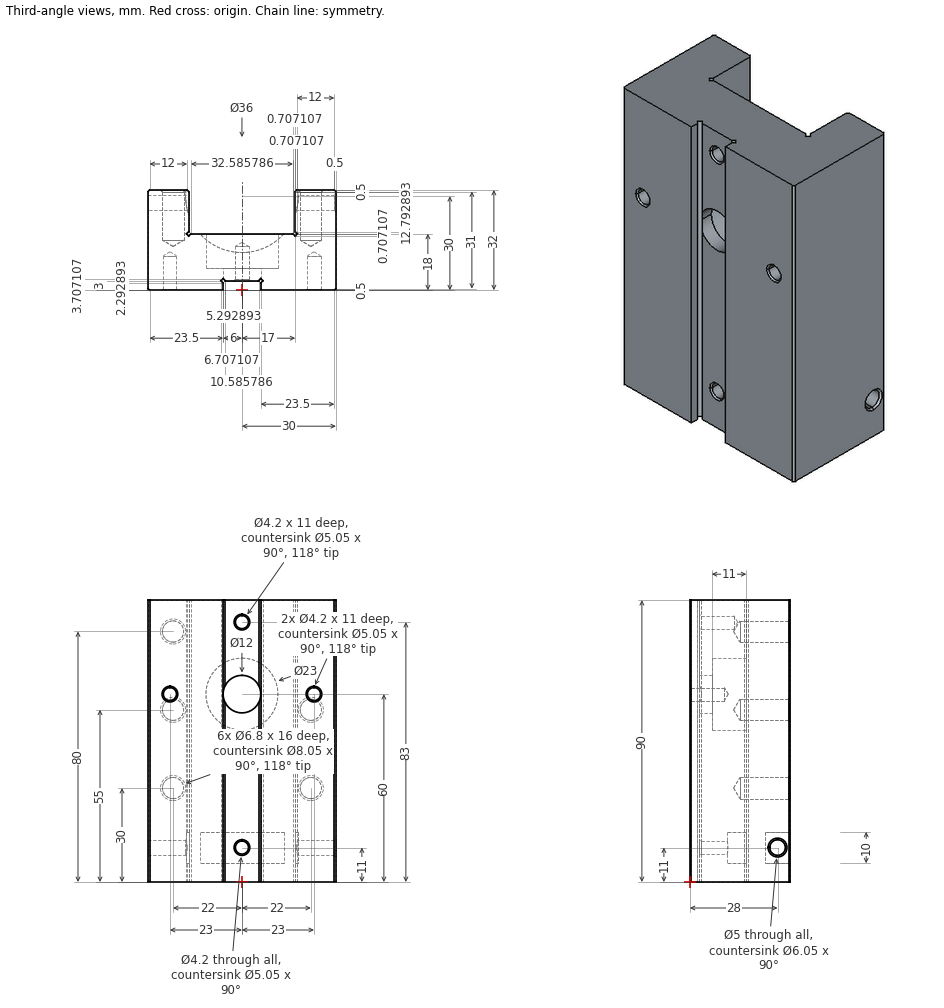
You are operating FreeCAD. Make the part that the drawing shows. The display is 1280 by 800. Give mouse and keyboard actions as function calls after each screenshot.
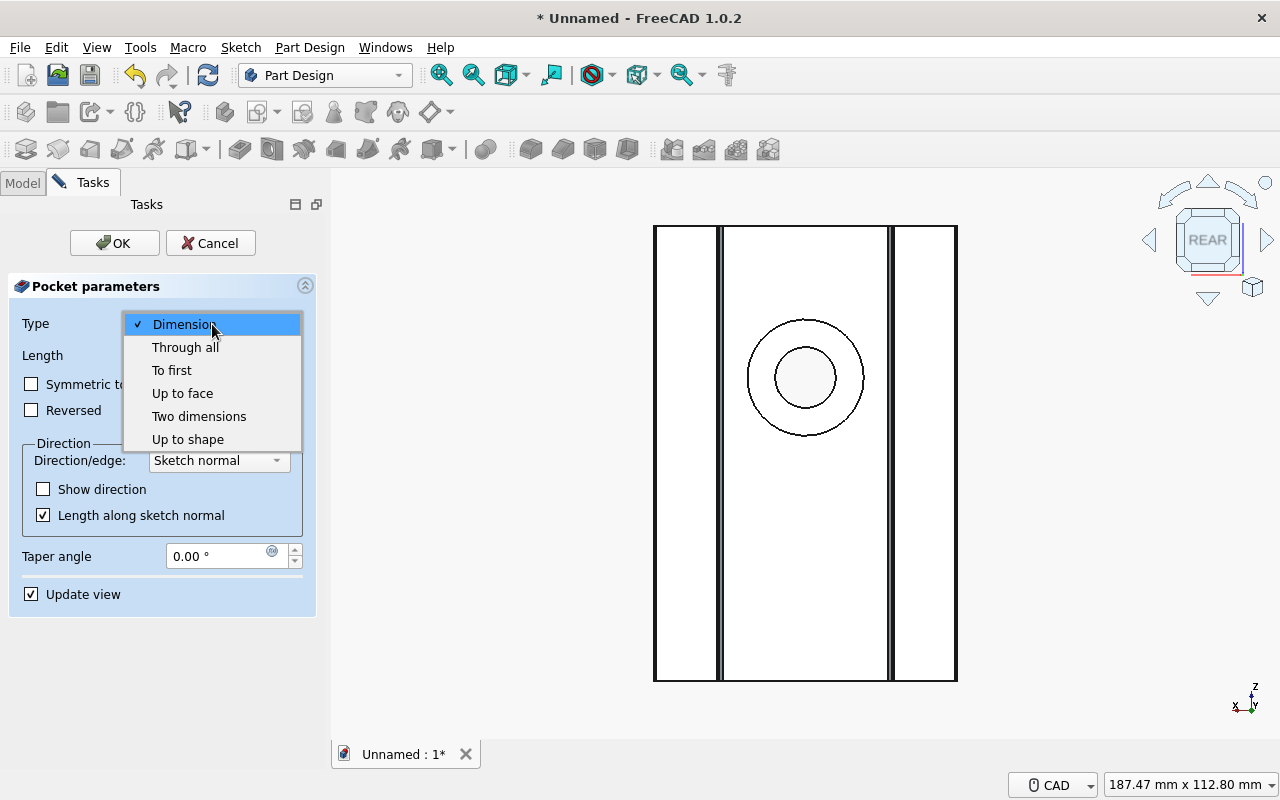
click(212, 348)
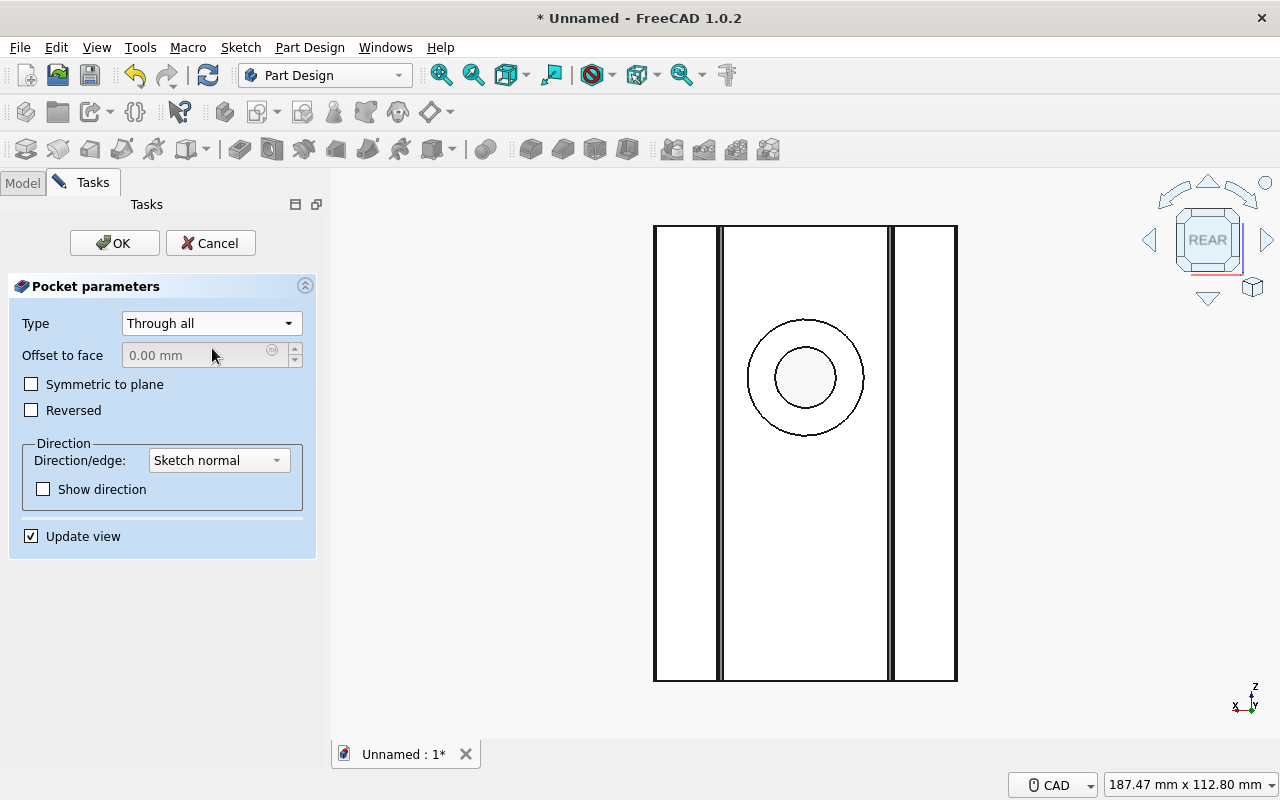
click(115, 243)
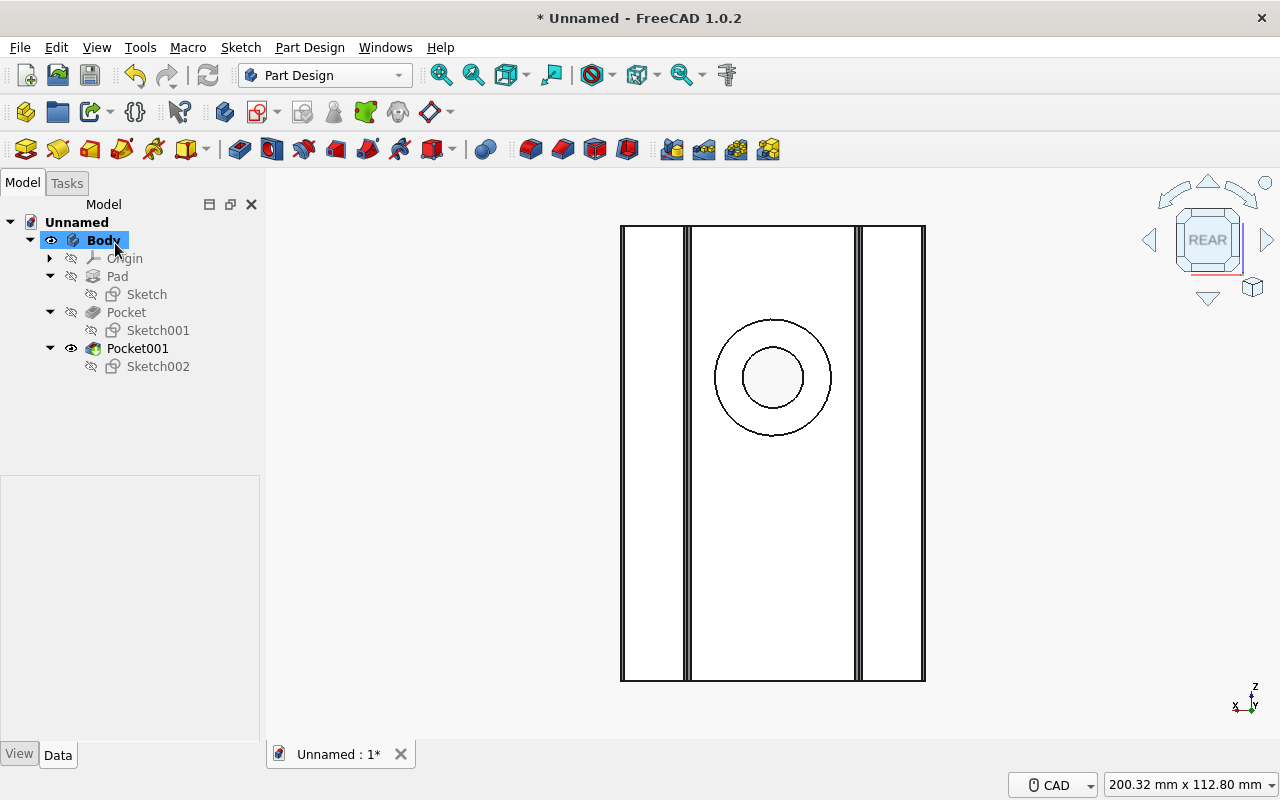
click(50, 258)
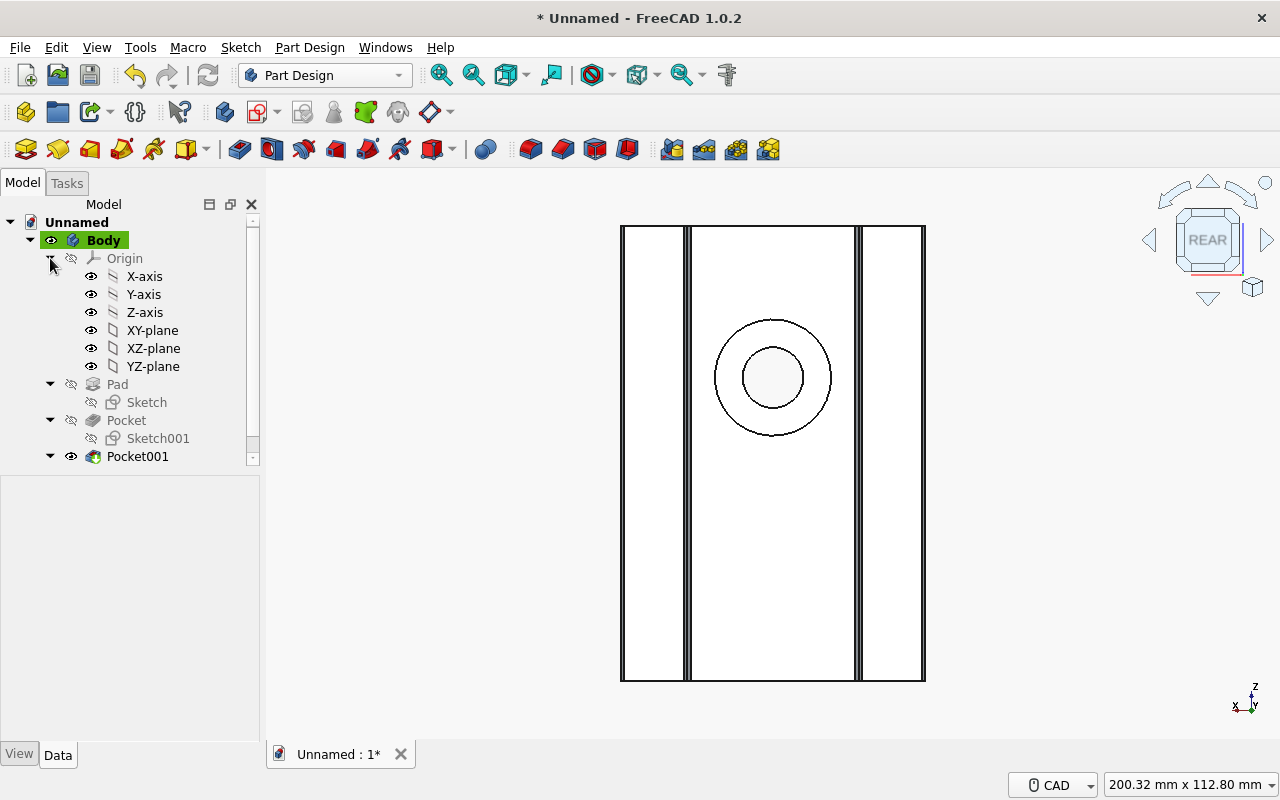
click(136, 330)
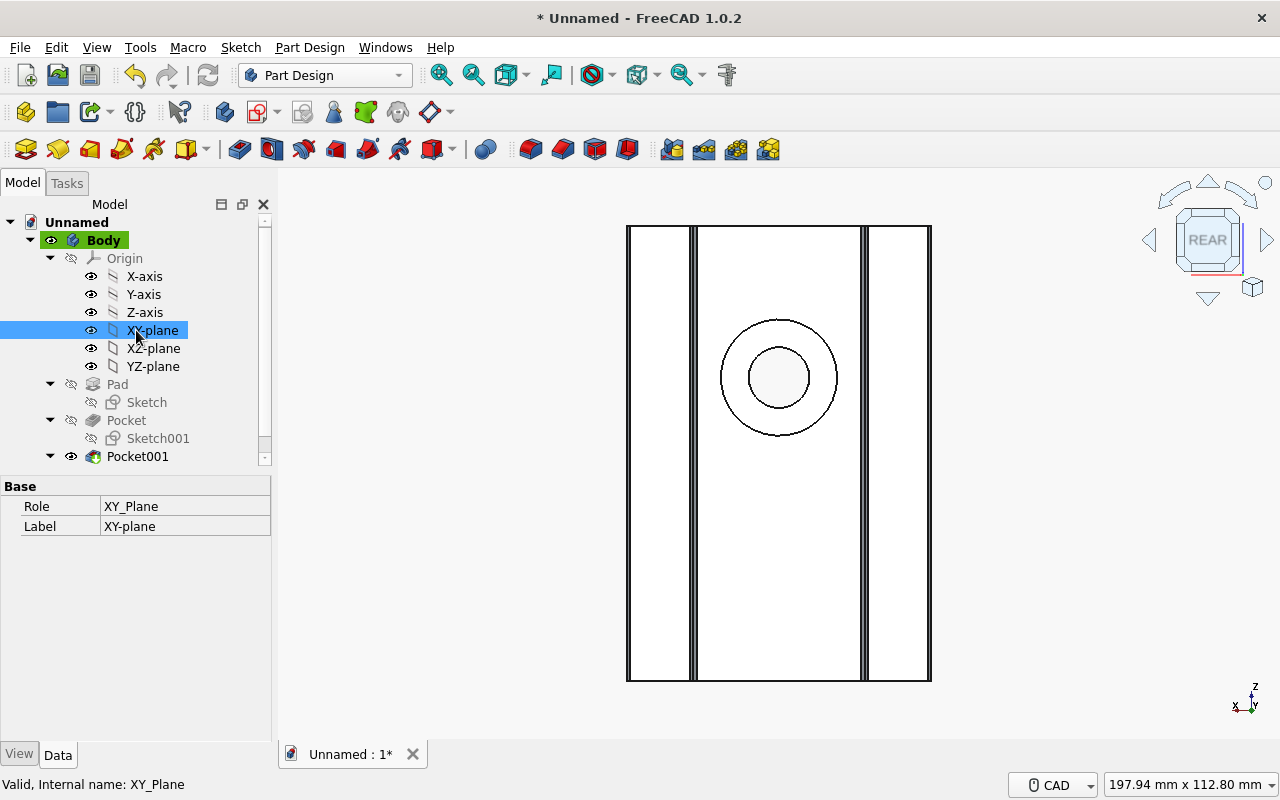
click(430, 112)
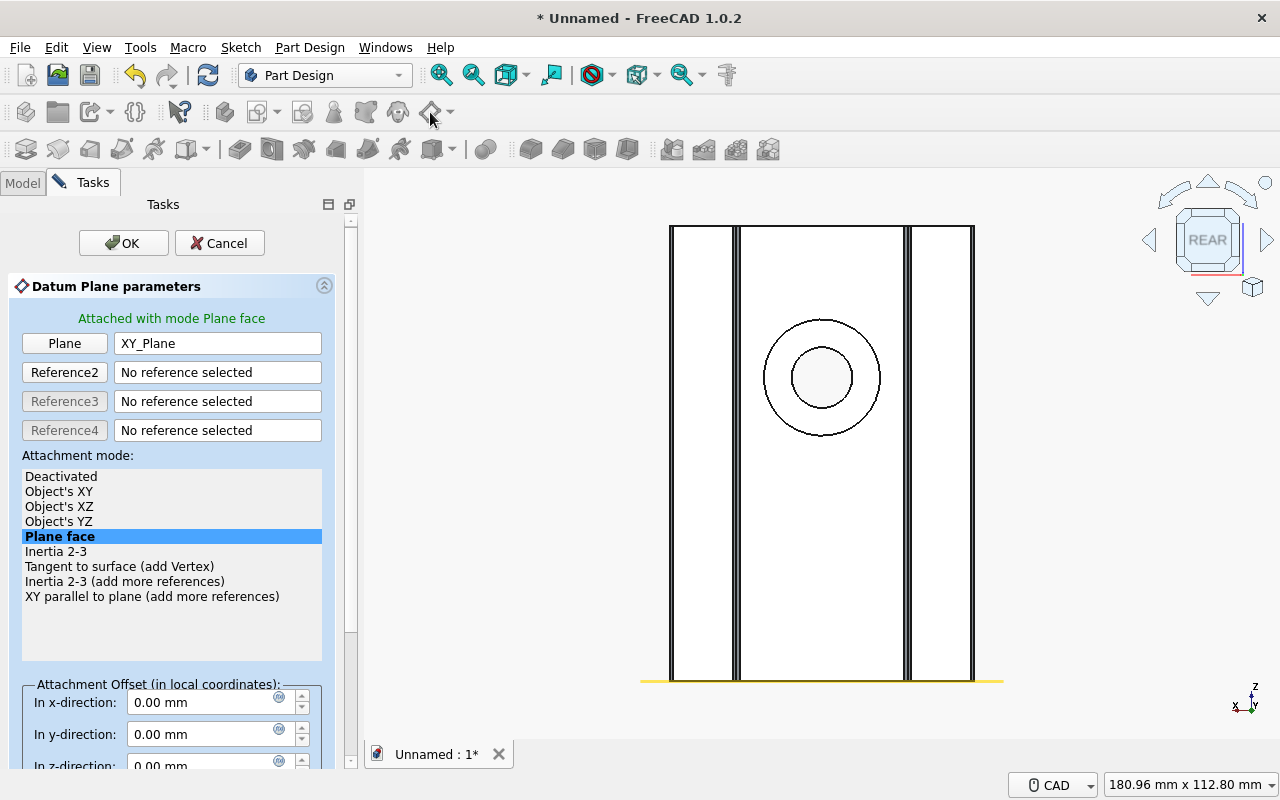
scroll(351, 491, down, 2)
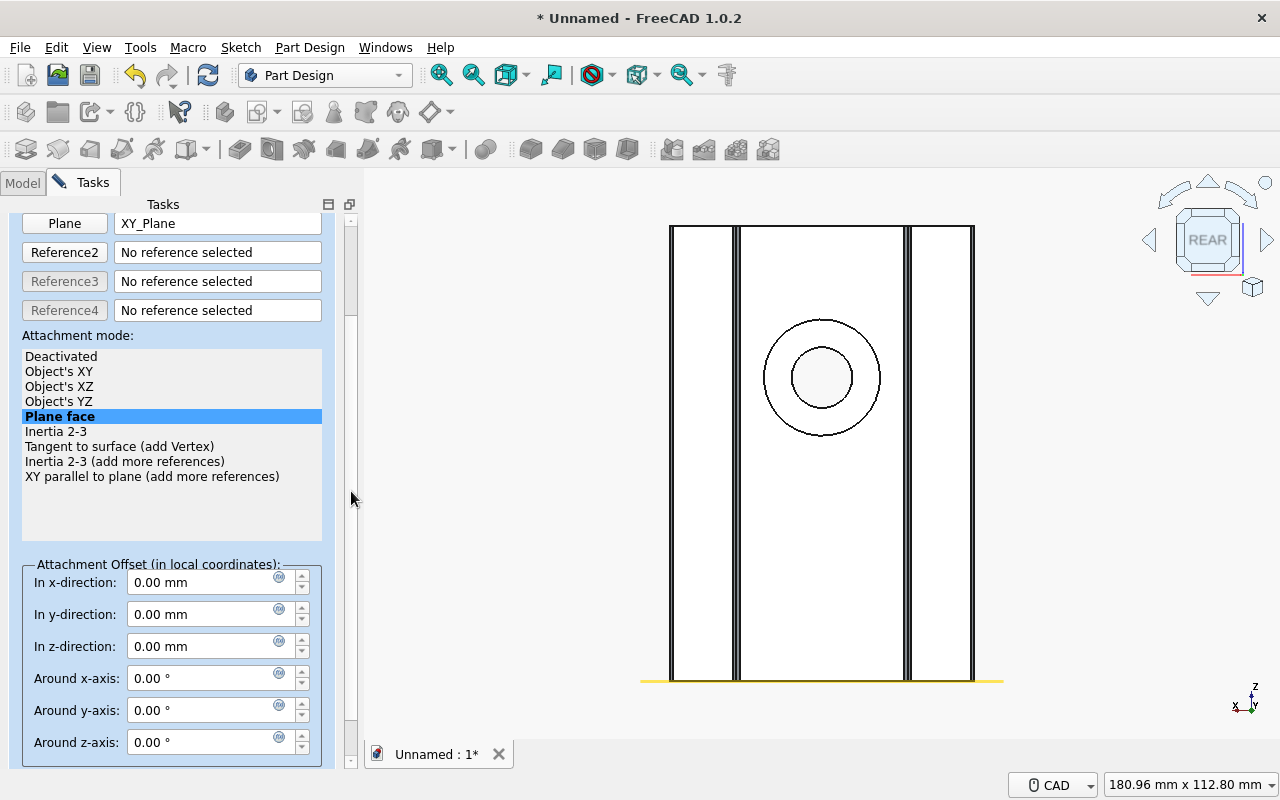
triple_click(210, 646)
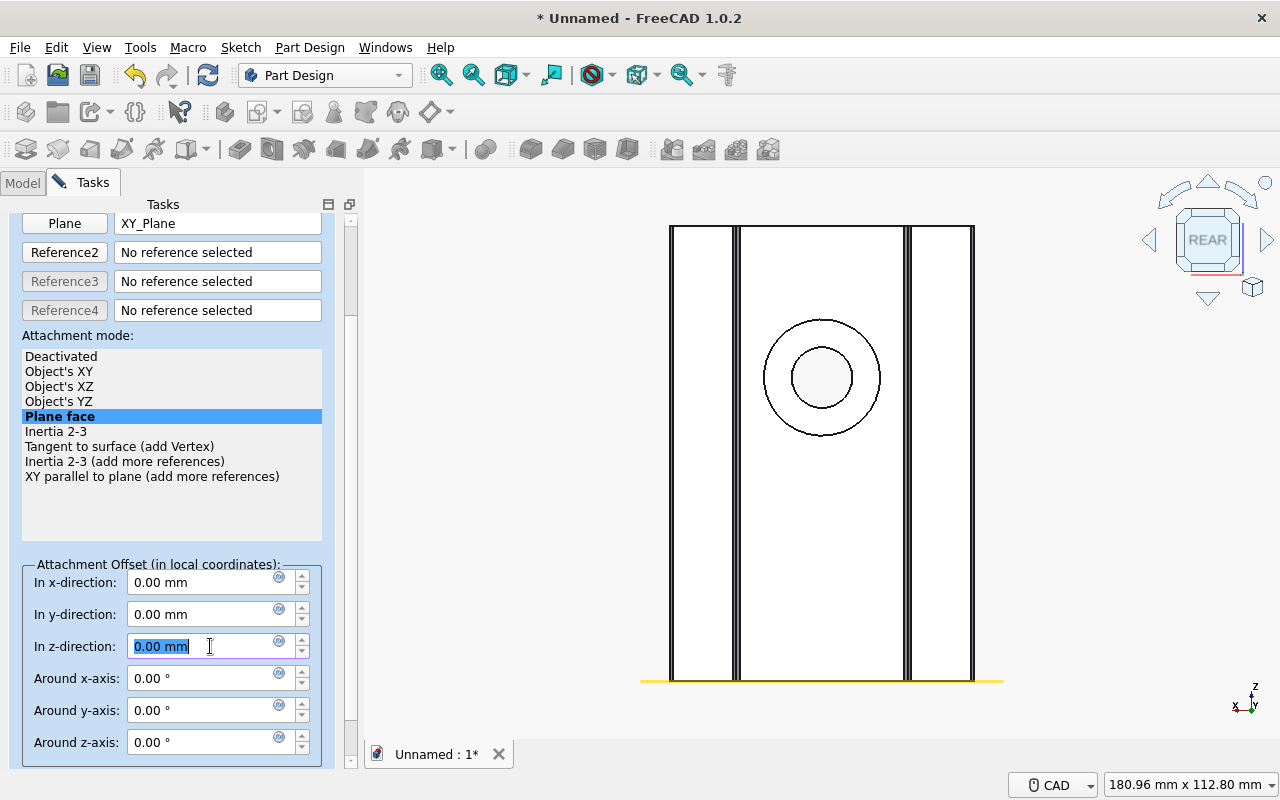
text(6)
key(Tab)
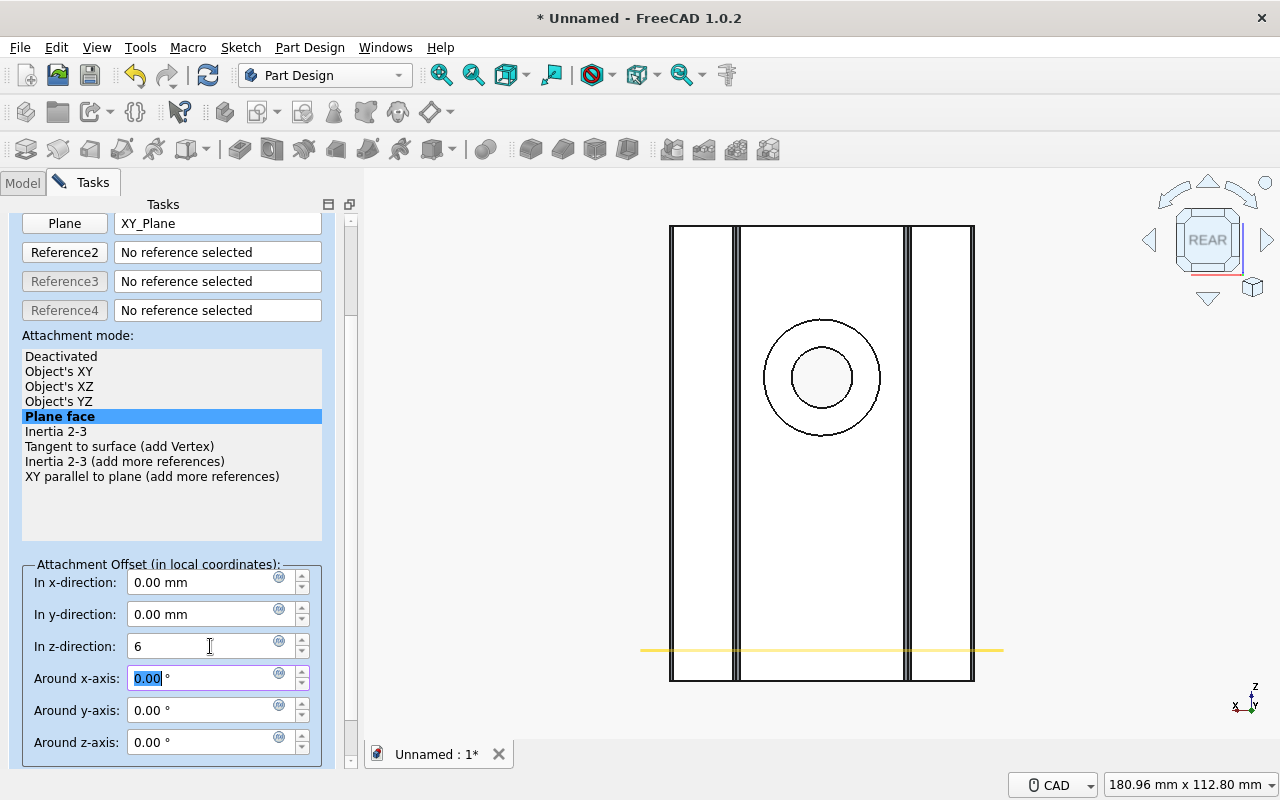
scroll(351, 491, up, 3)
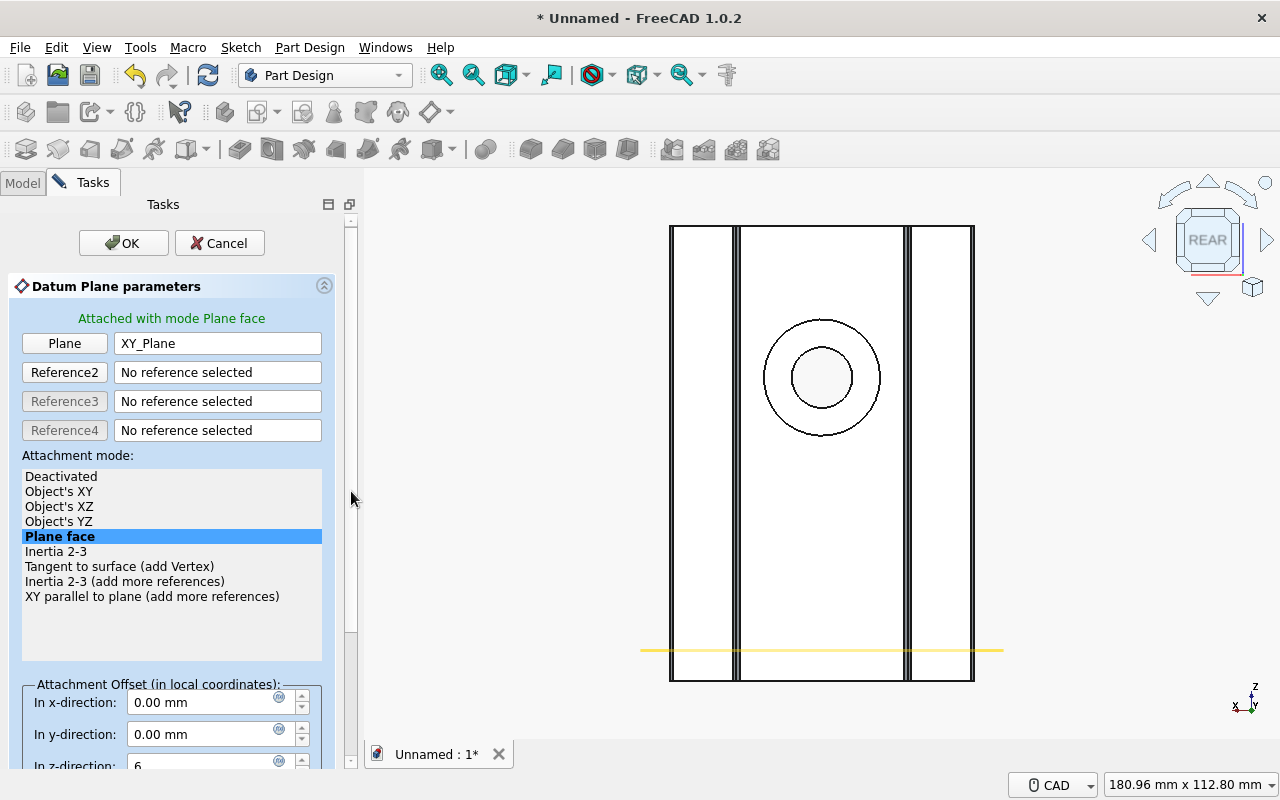
click(124, 243)